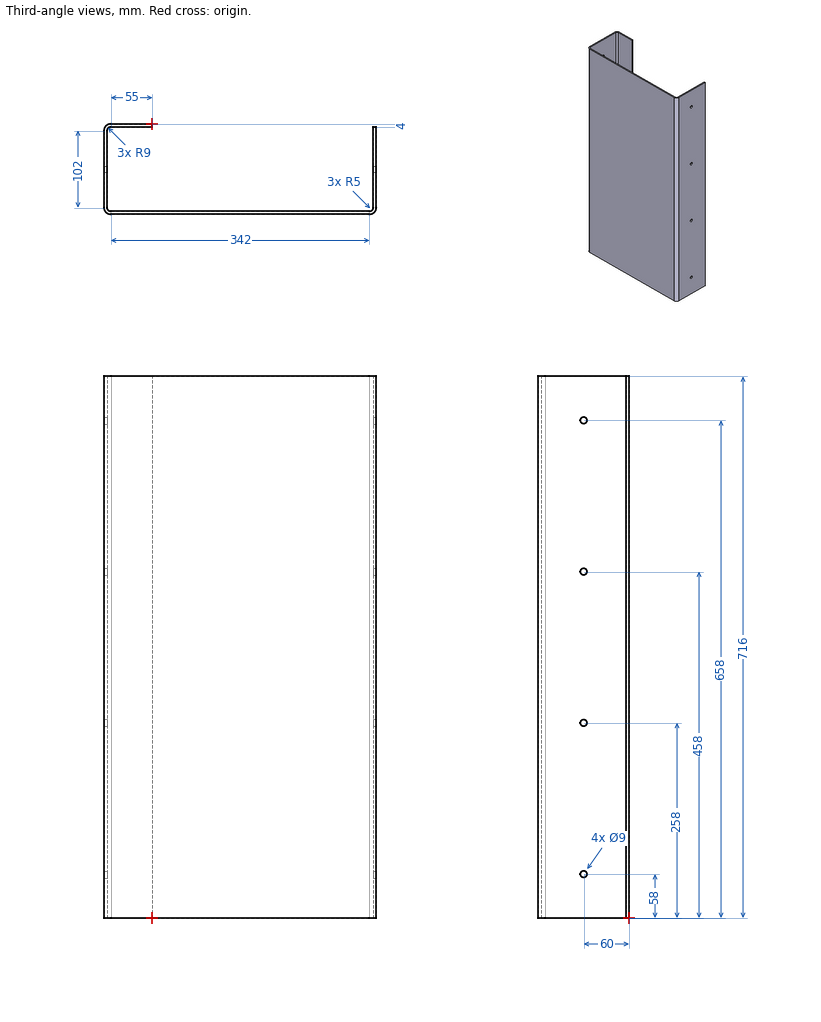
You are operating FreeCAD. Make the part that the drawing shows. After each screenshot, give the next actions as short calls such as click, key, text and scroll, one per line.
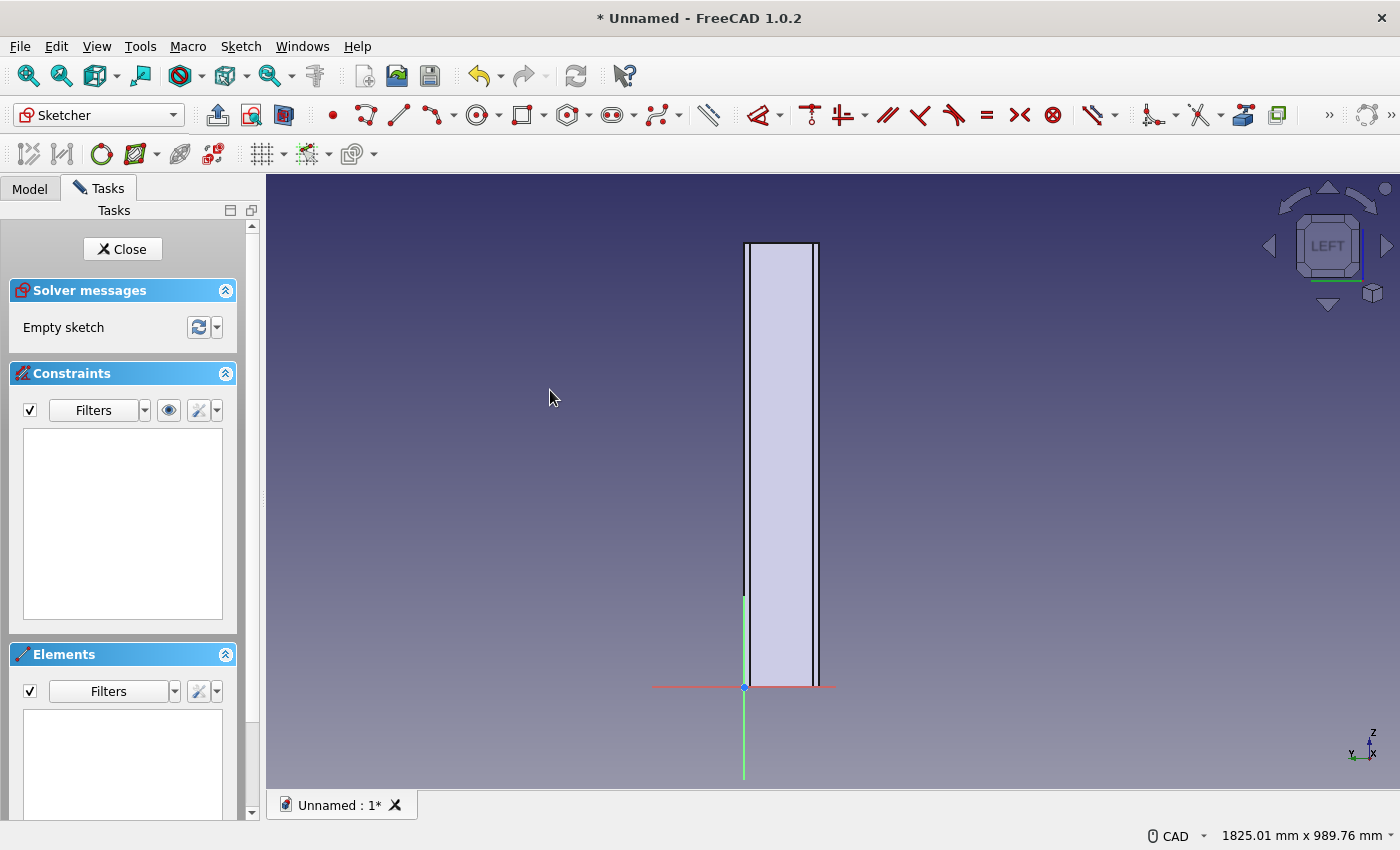
click(476, 116)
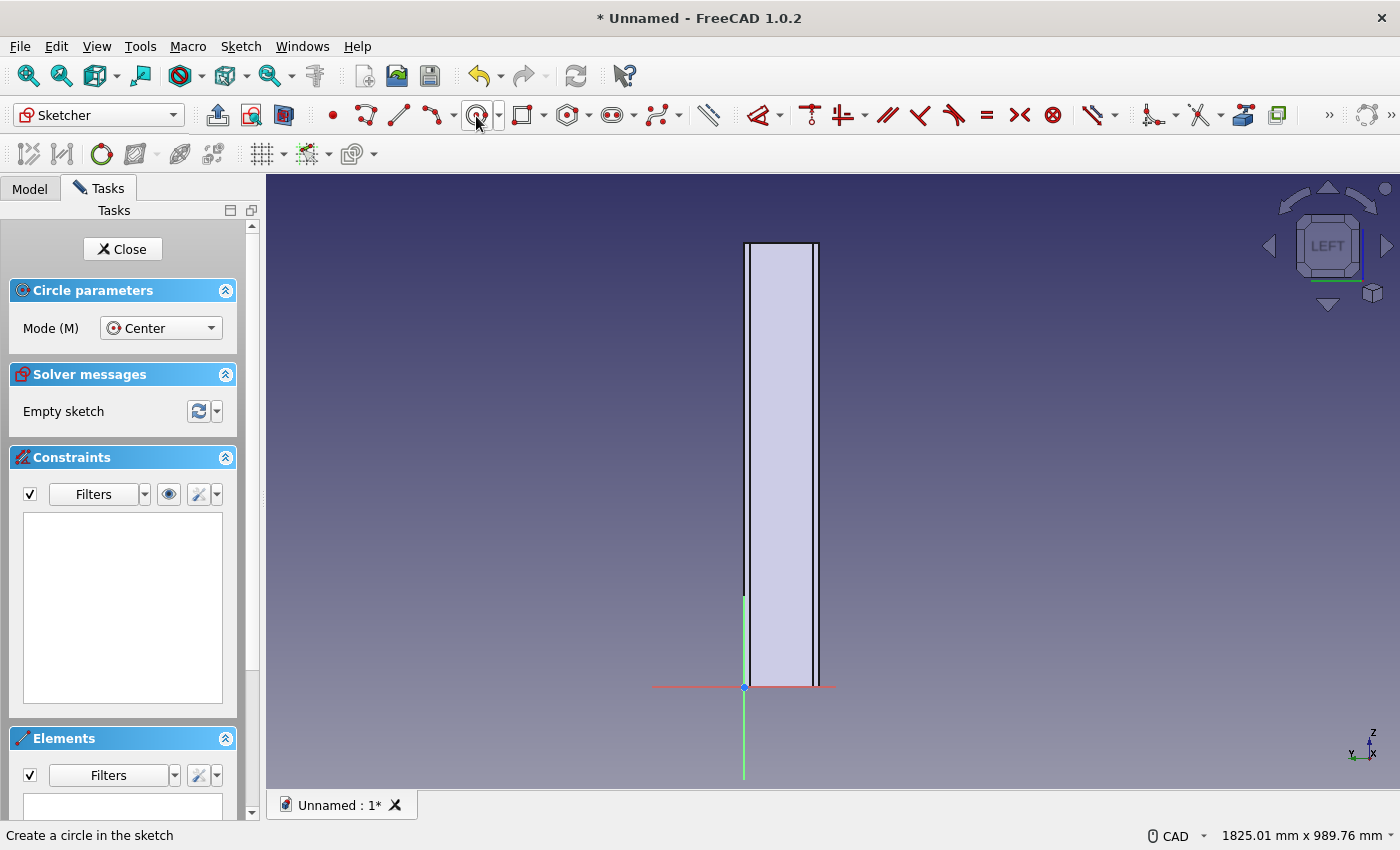
scroll(782, 651, up, 11)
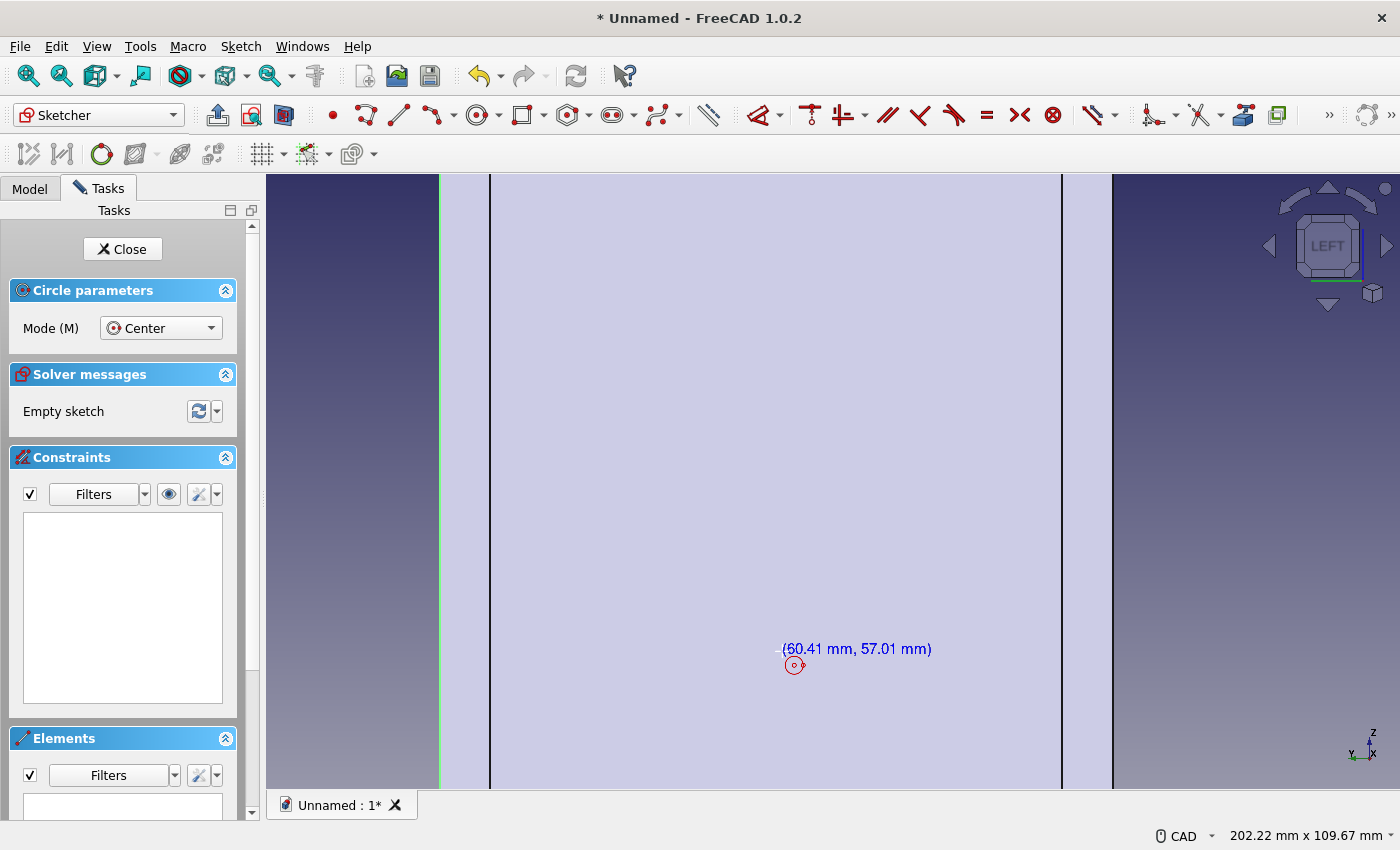
scroll(782, 652, down, 11)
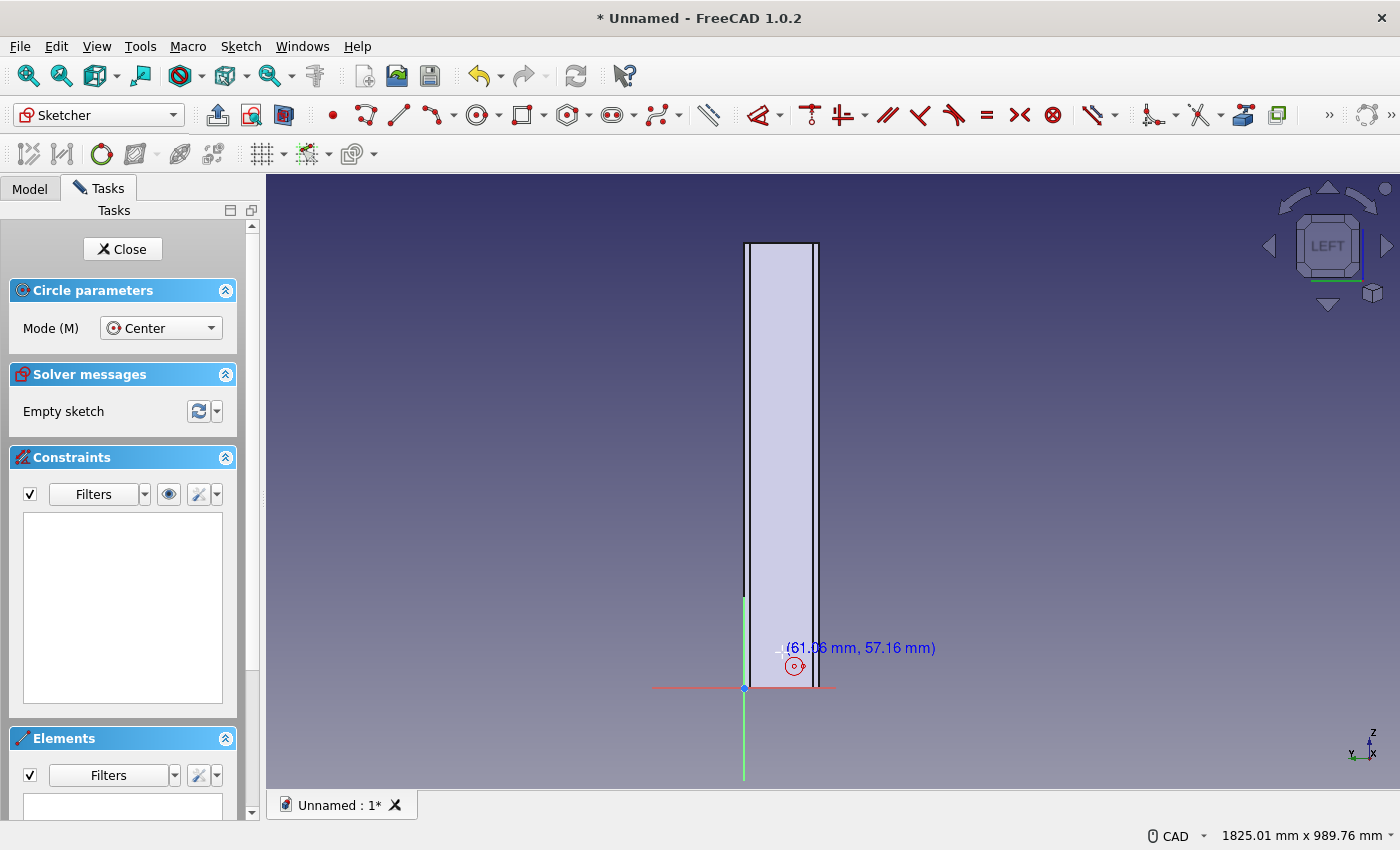
click(782, 652)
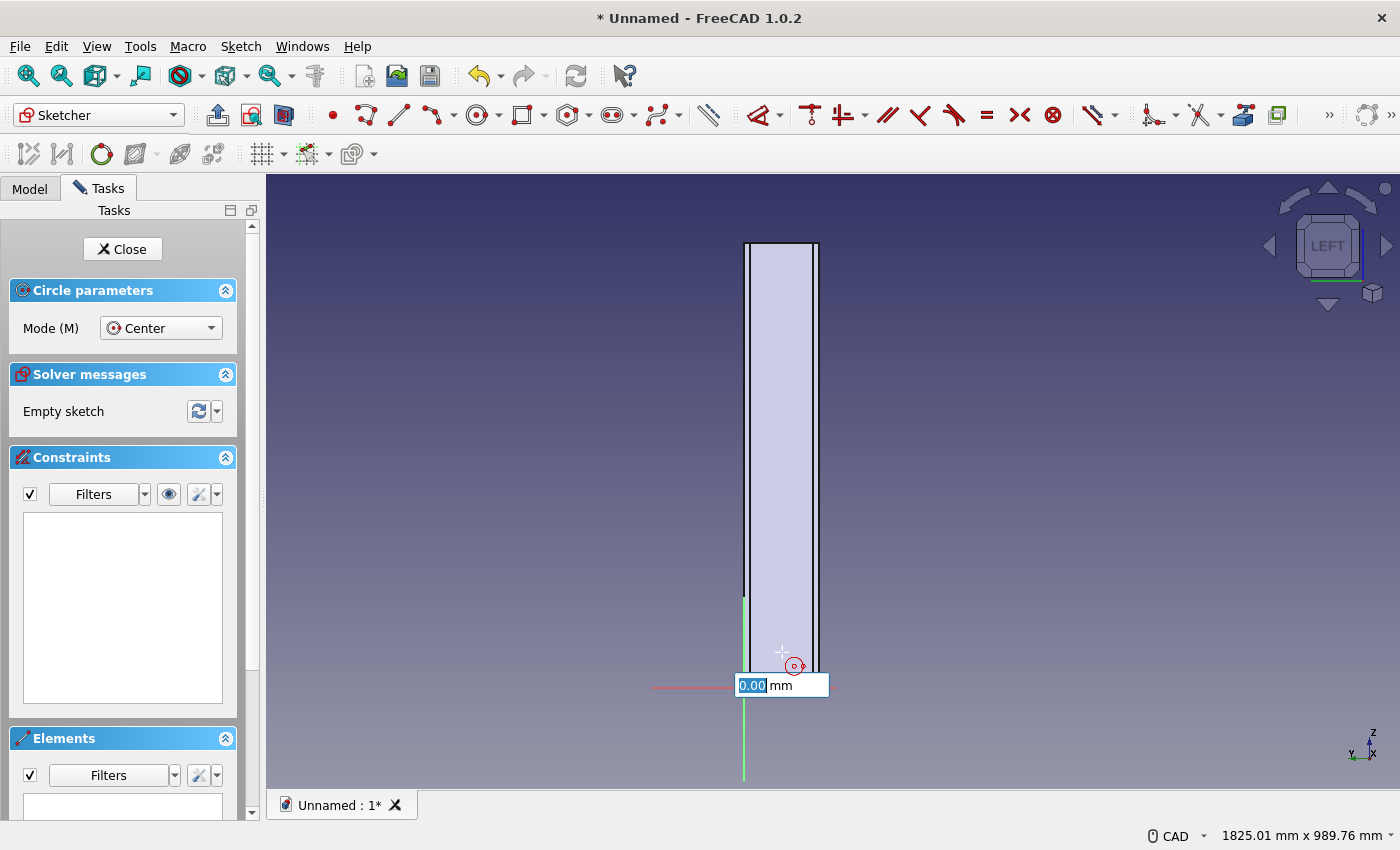
scroll(784, 650, up, 9)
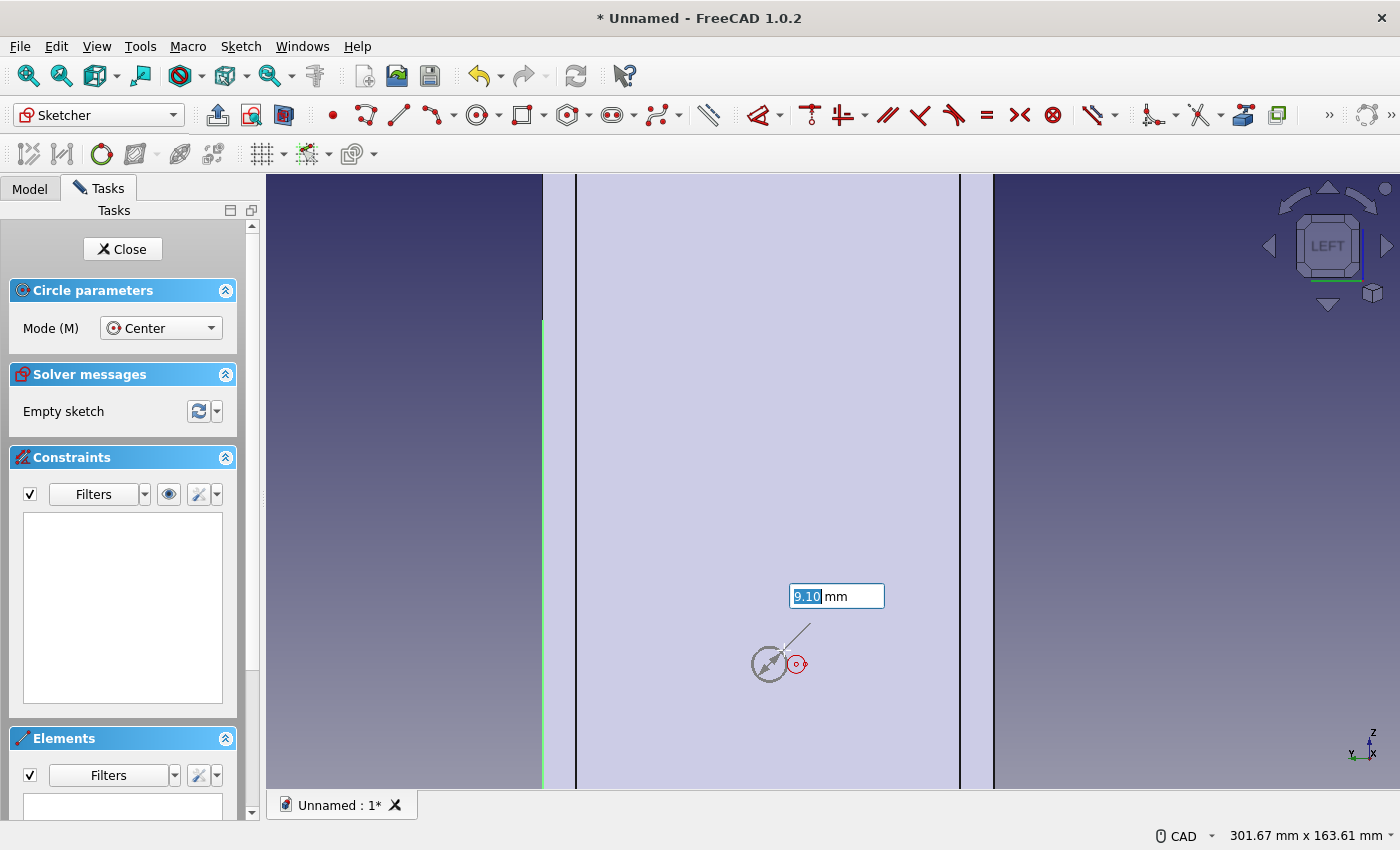
click(780, 648)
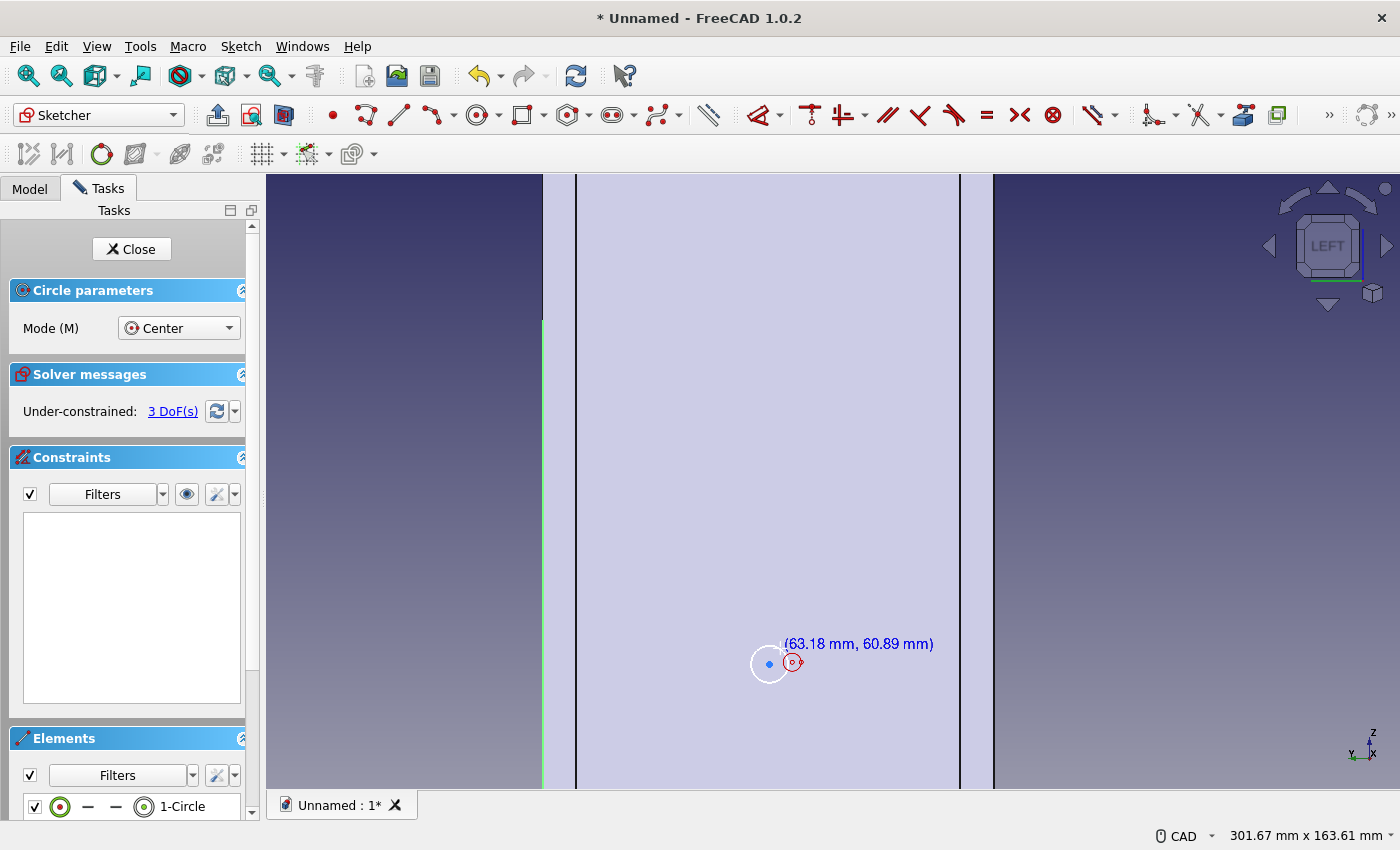
scroll(784, 650, down, 9)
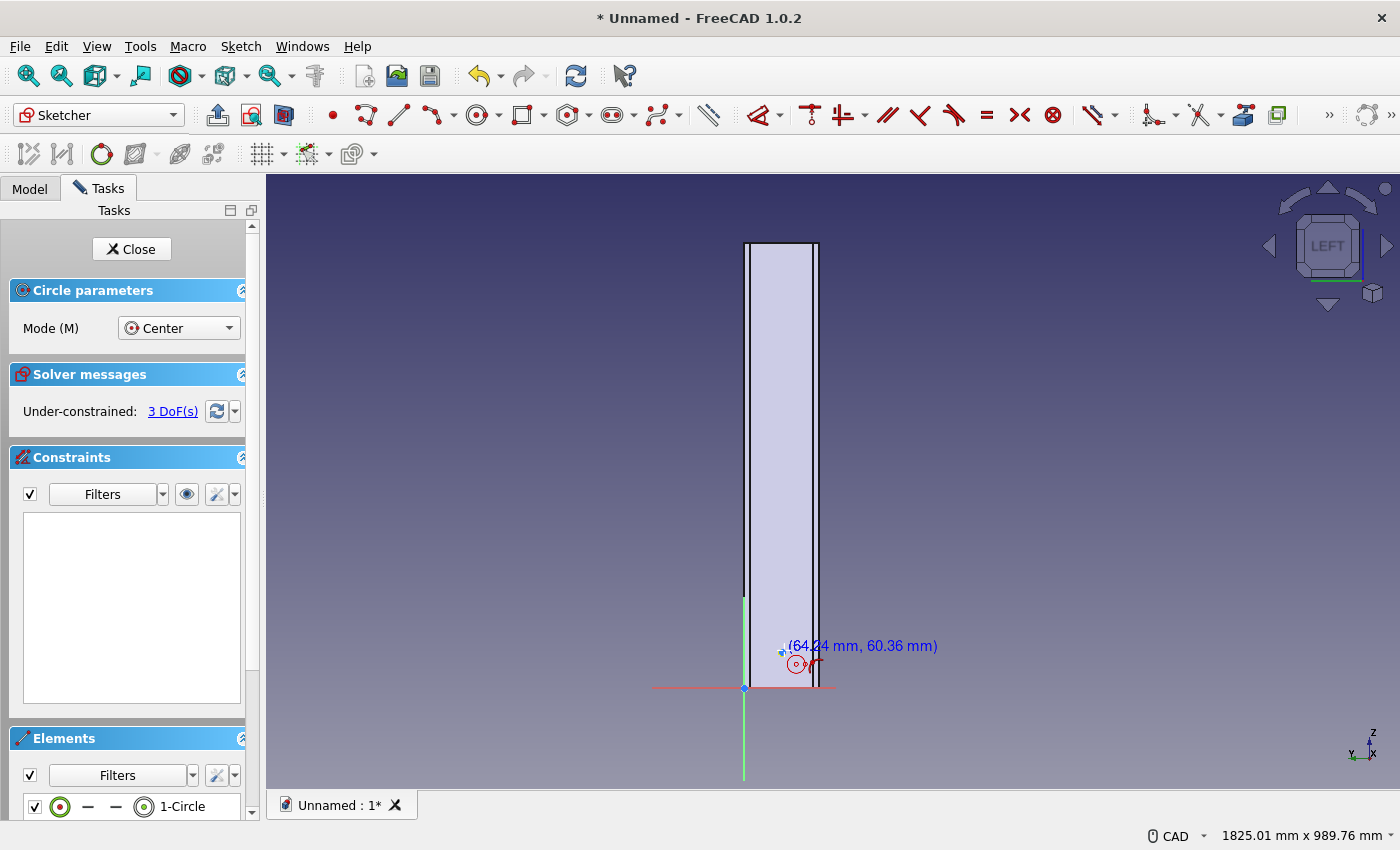
scroll(782, 528, up, 11)